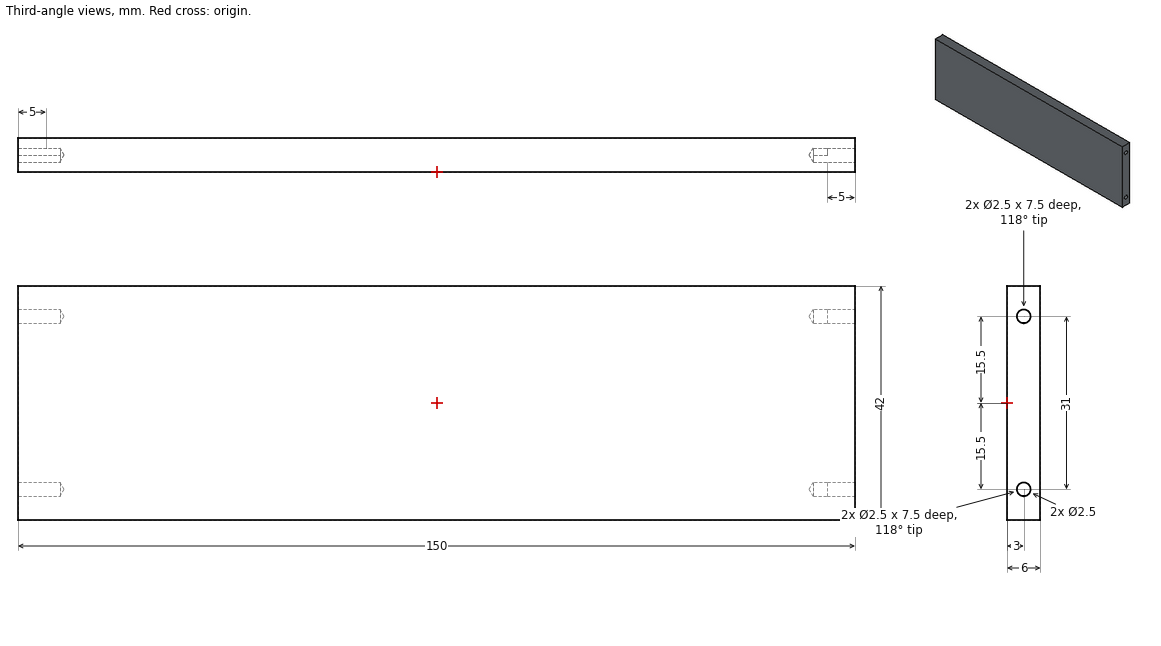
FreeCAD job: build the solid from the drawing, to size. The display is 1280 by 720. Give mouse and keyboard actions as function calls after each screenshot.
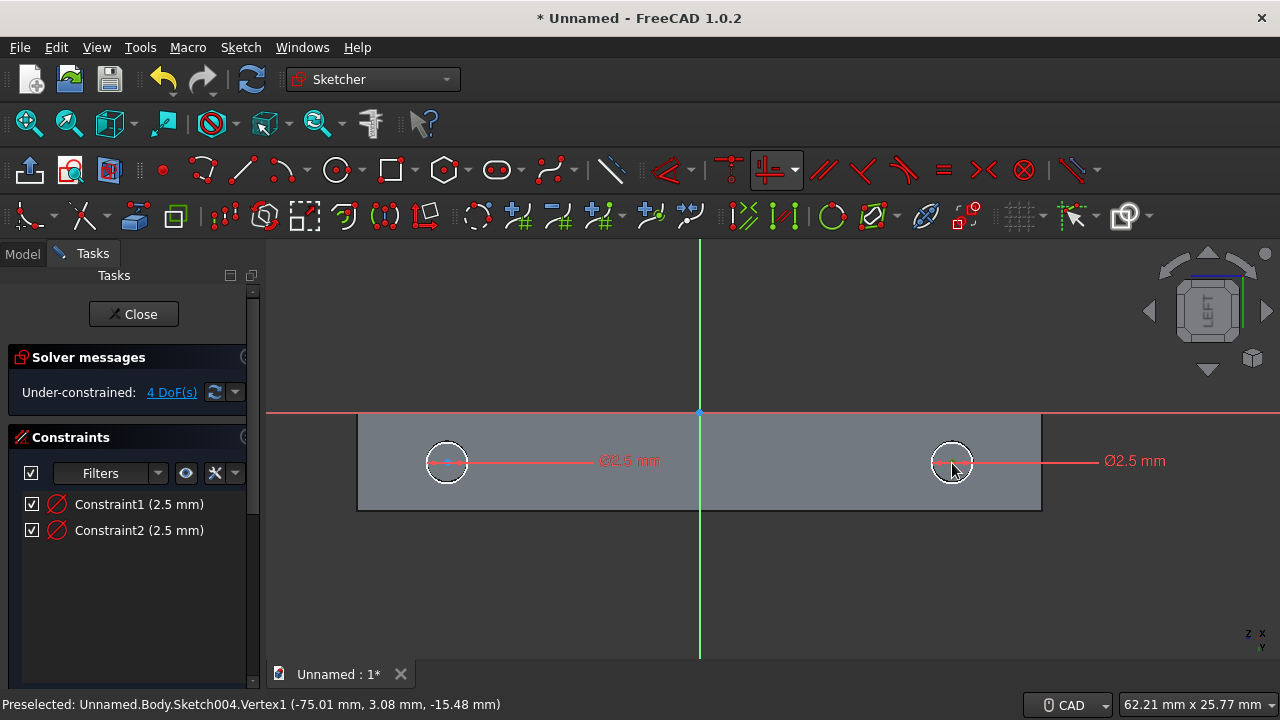
click(447, 463)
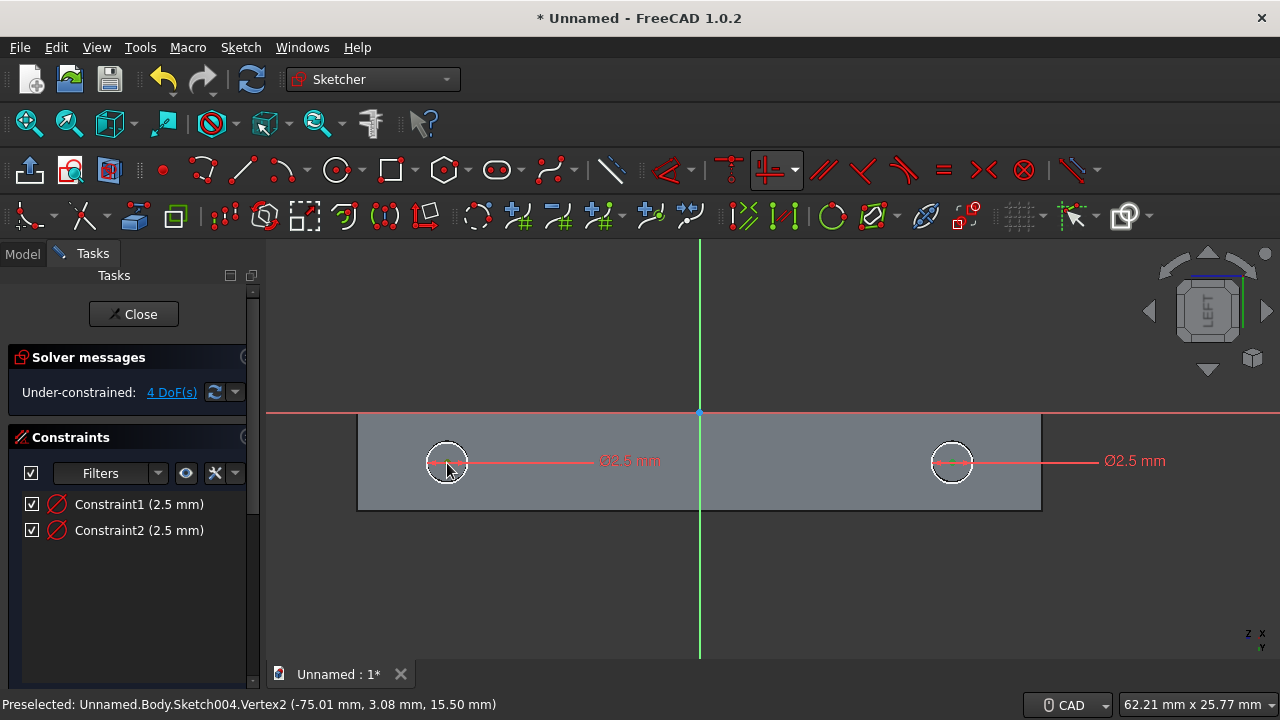
click(798, 170)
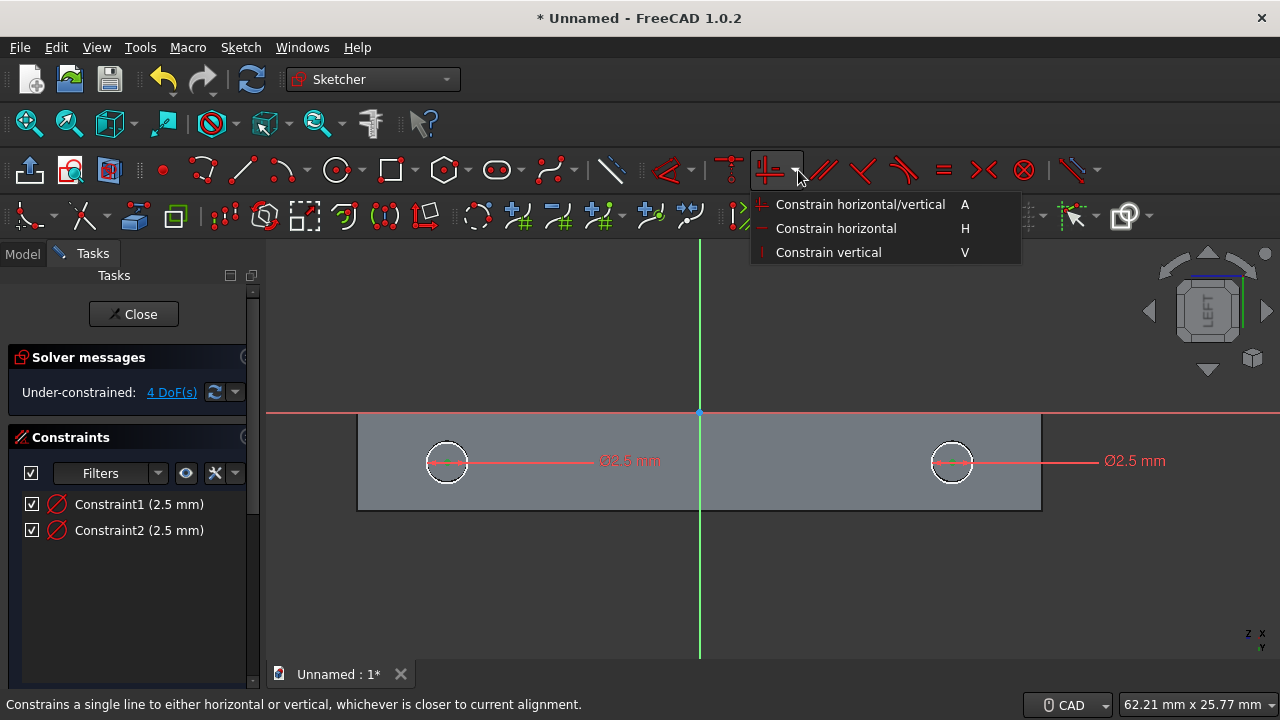
click(886, 228)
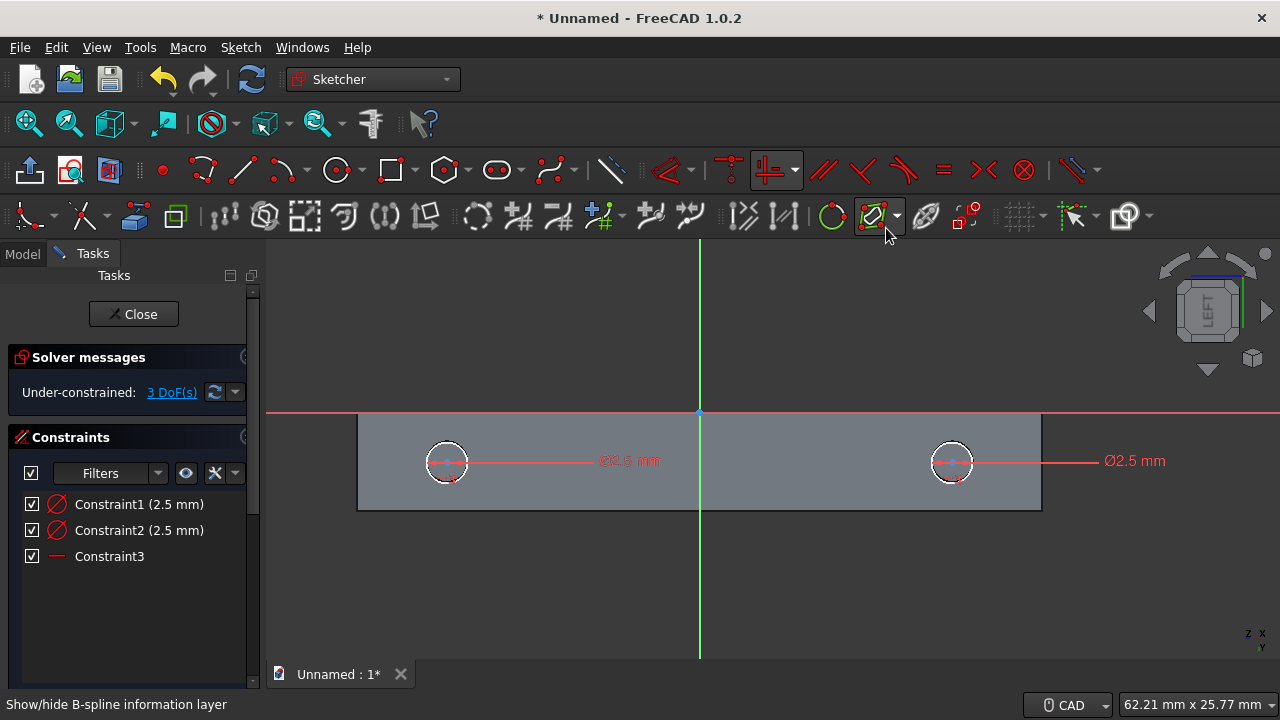
click(666, 170)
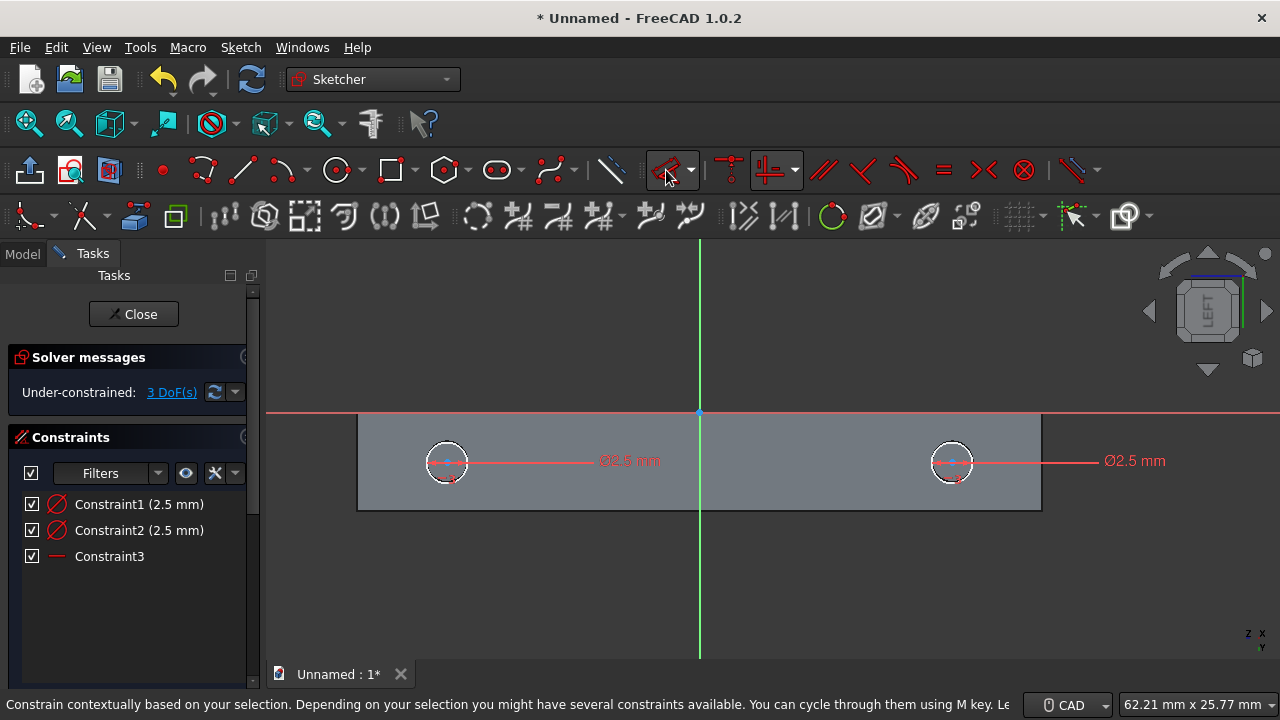
click(952, 463)
click(986, 438)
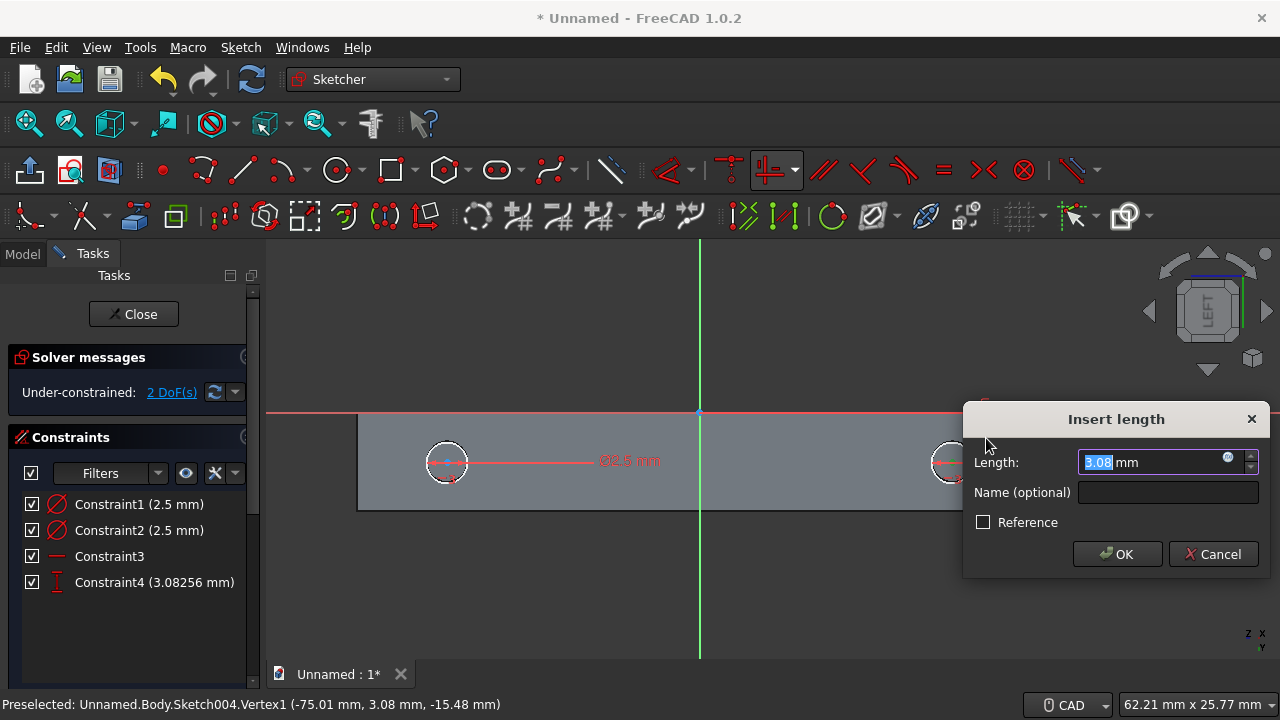
text(3)
key(Return)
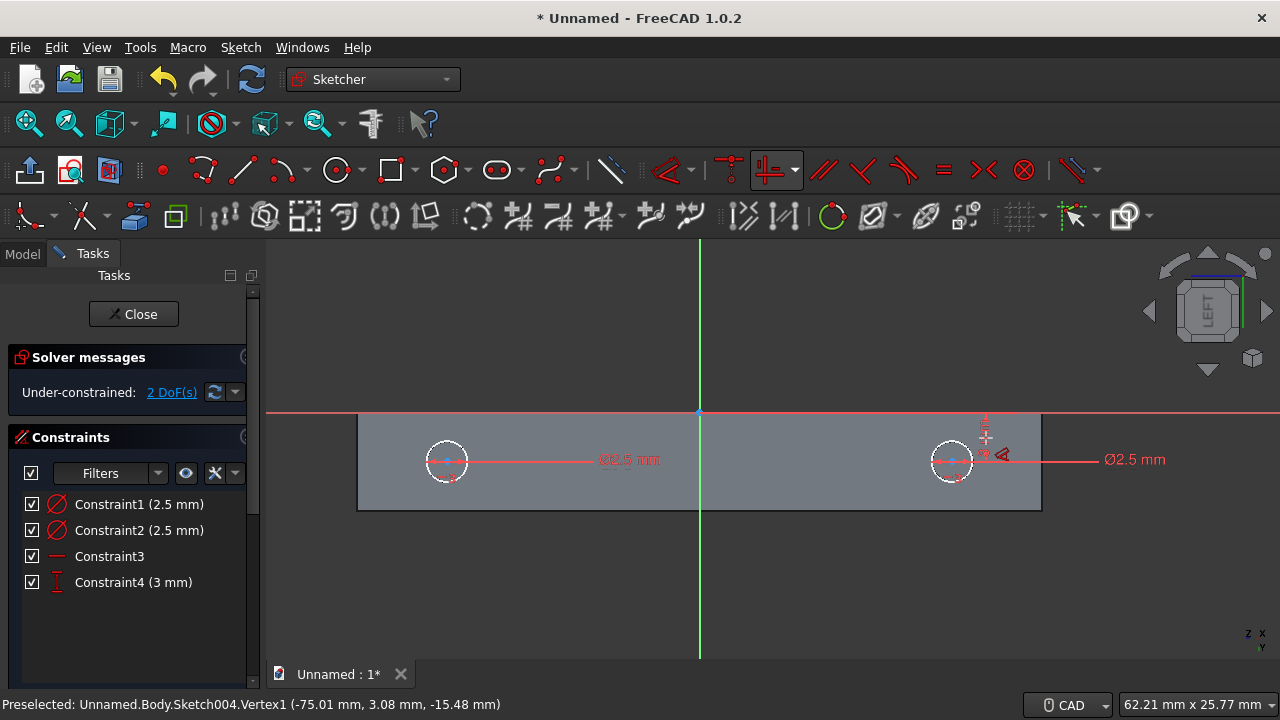
click(952, 462)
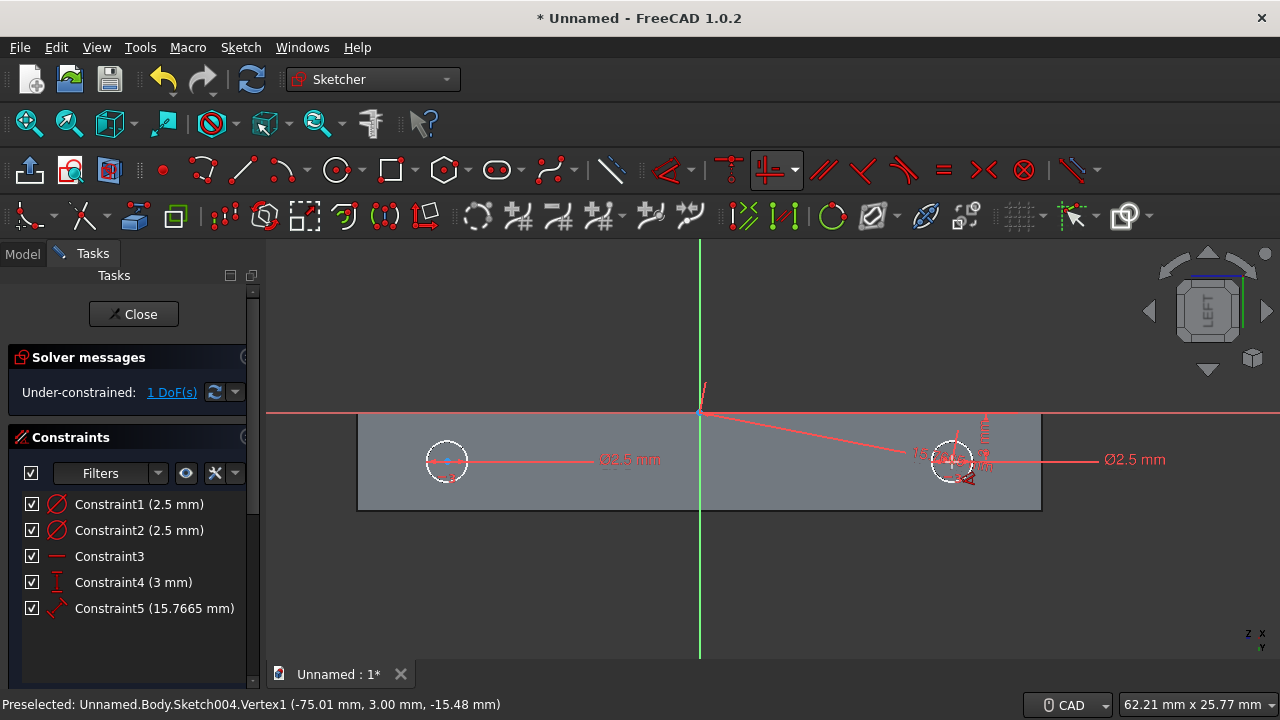
click(447, 462)
click(583, 496)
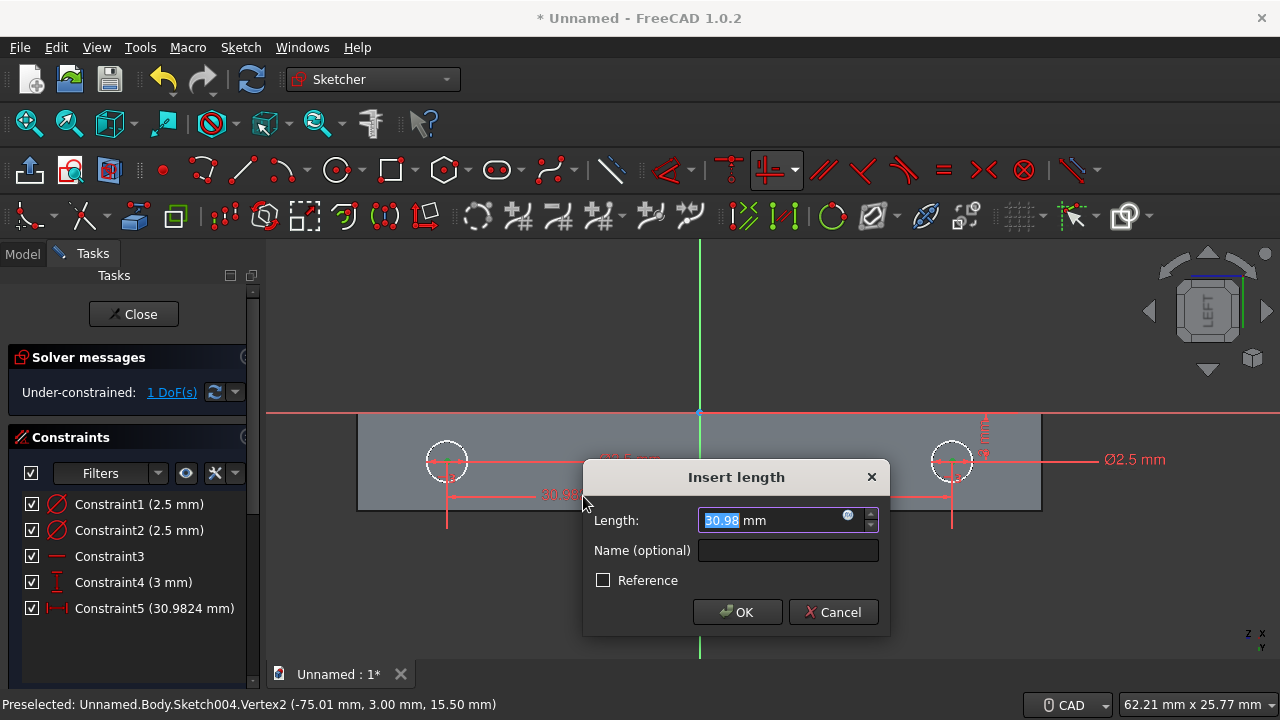
text(31)
key(Return)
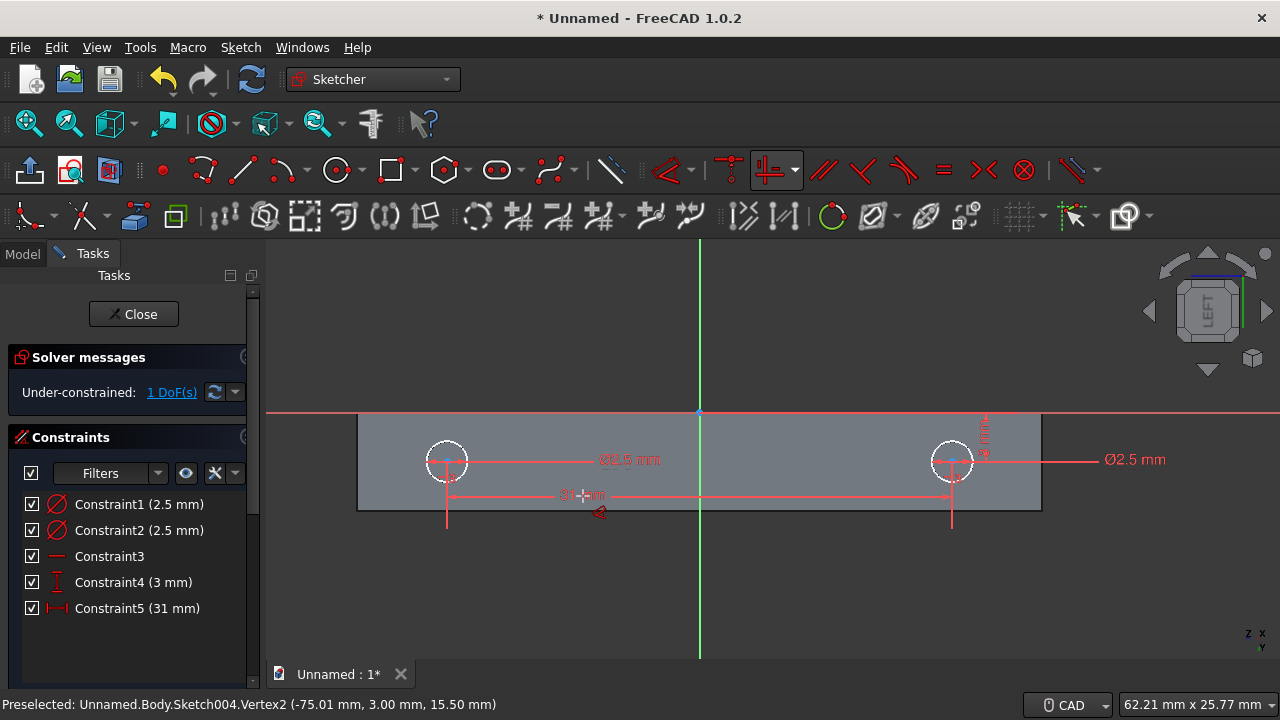
click(952, 462)
click(826, 379)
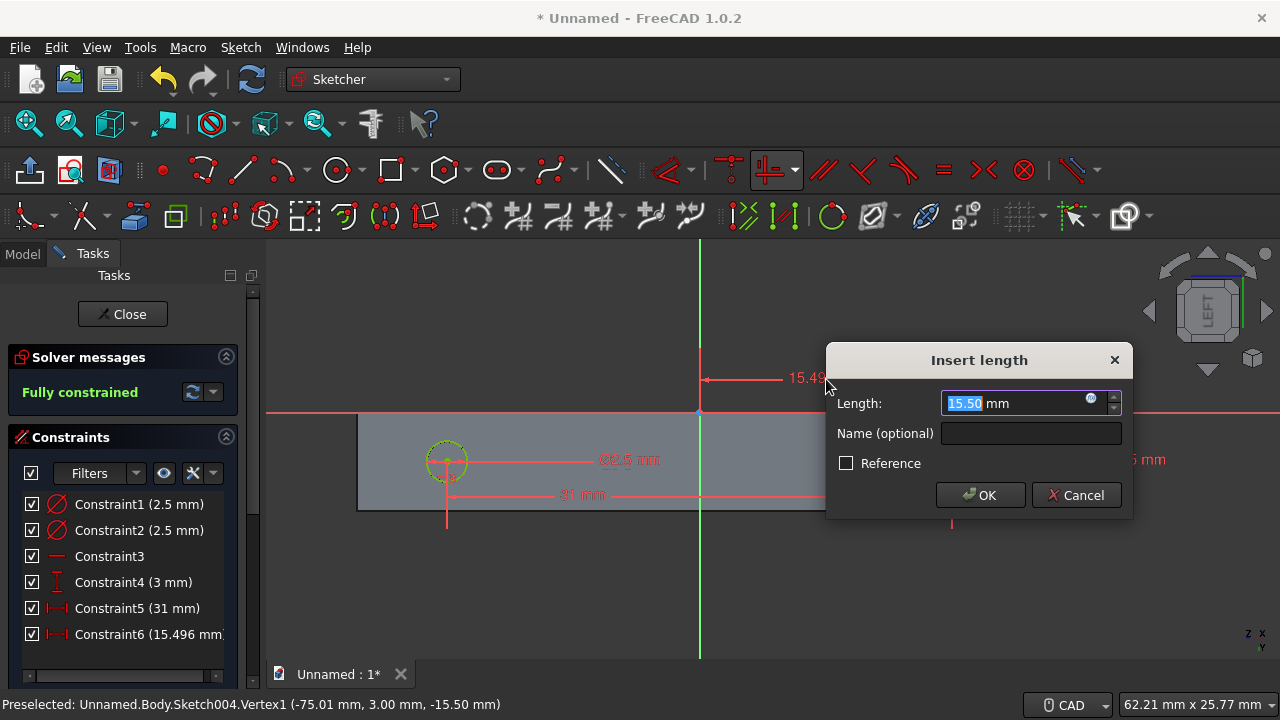
text(15.5)
key(Return)
key(Escape)